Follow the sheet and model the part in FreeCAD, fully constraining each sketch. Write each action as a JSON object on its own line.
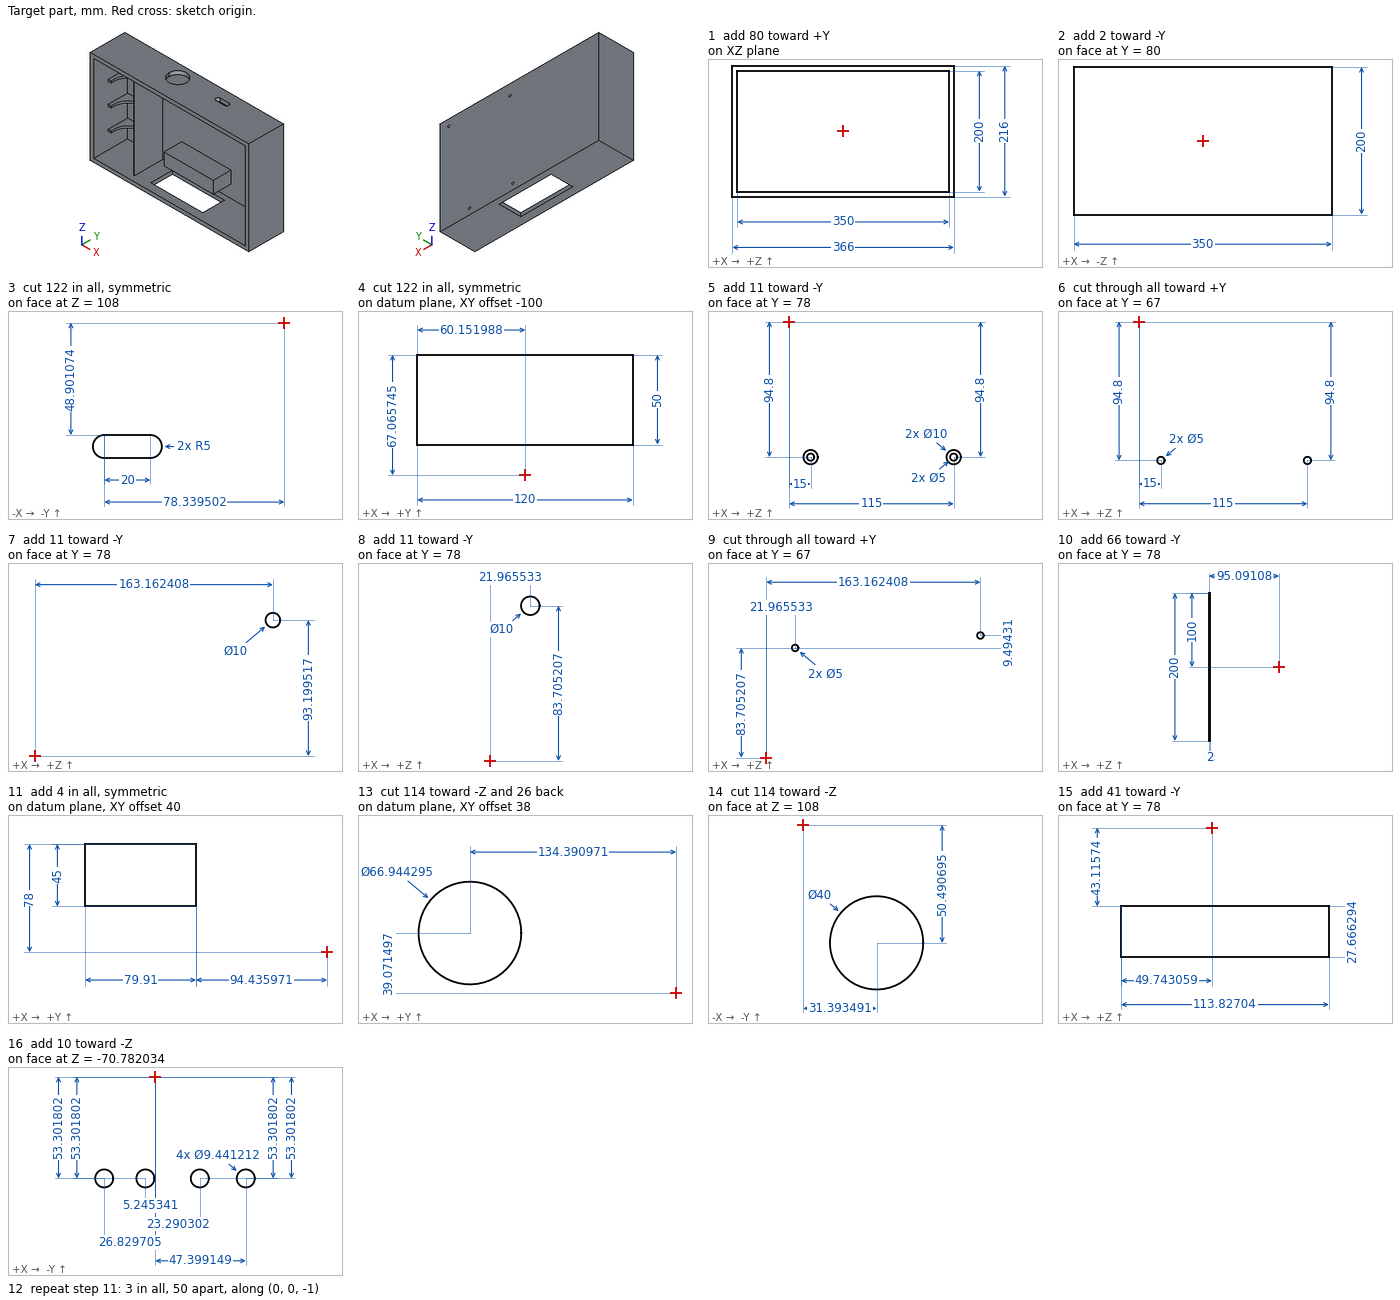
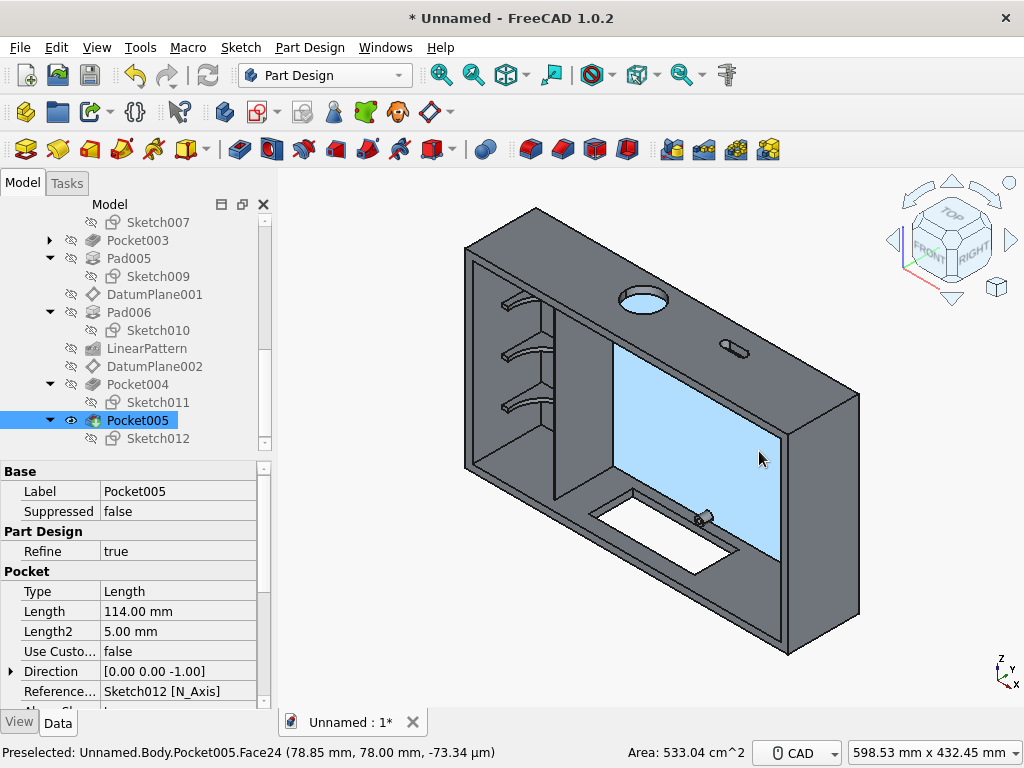
{"action": "left_click", "coordinate": [258, 112]}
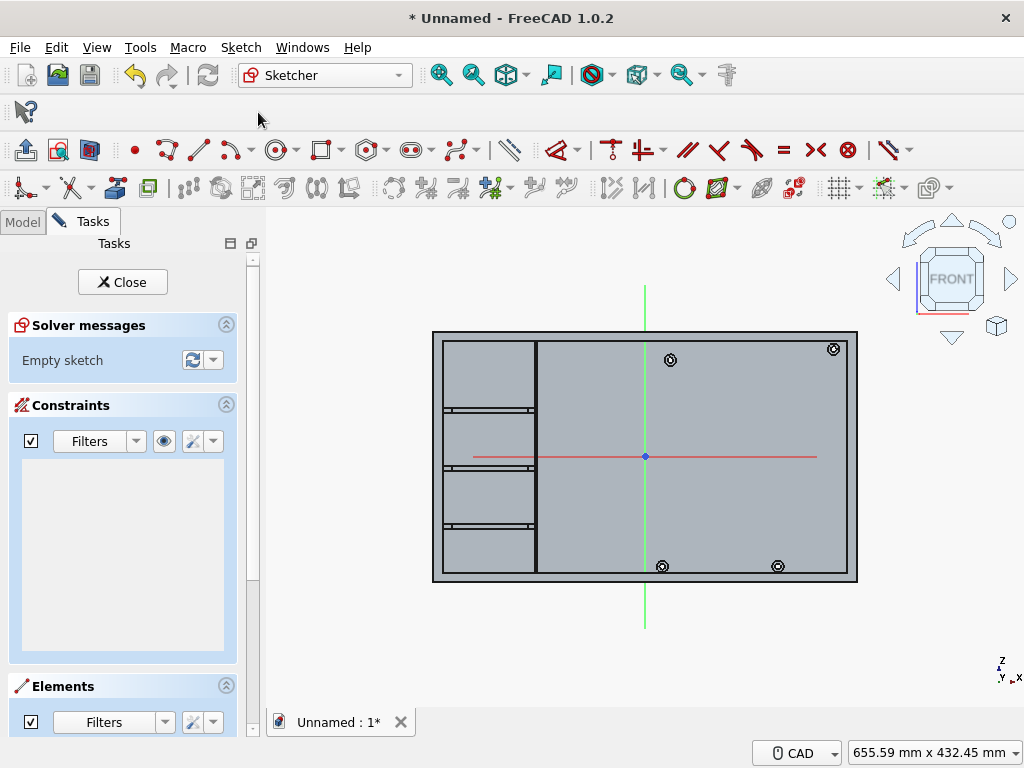
{"action": "key", "text": "q s"}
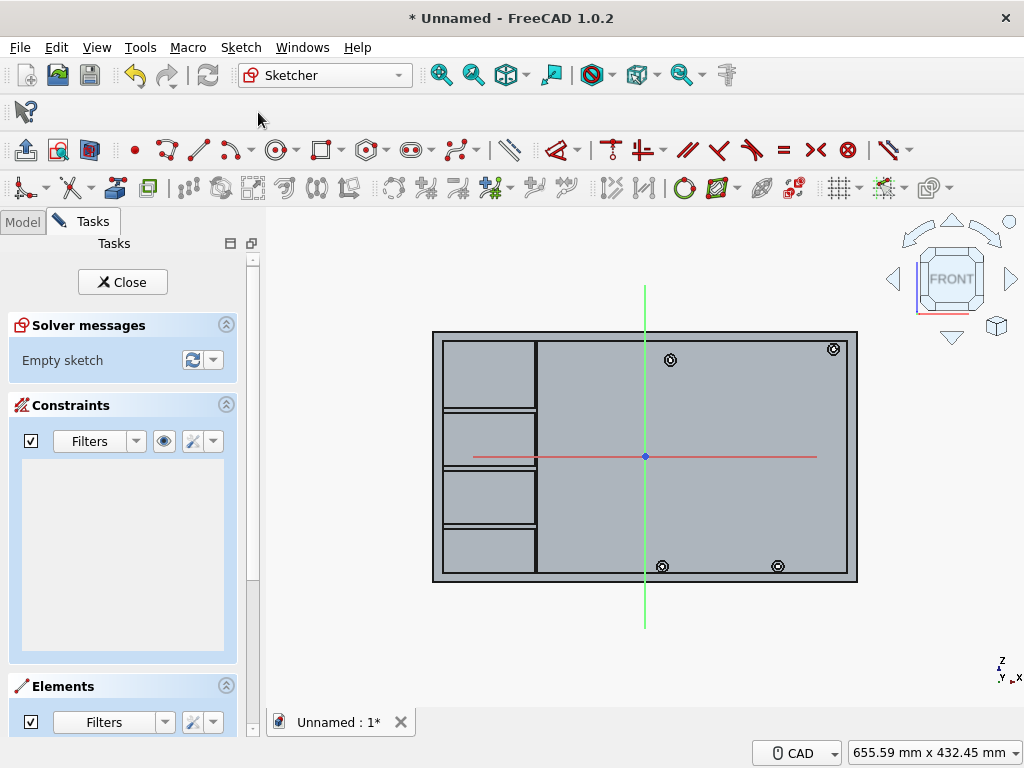
{"action": "scroll", "coordinate": [686, 516], "scroll_direction": "up", "scroll_amount": 6}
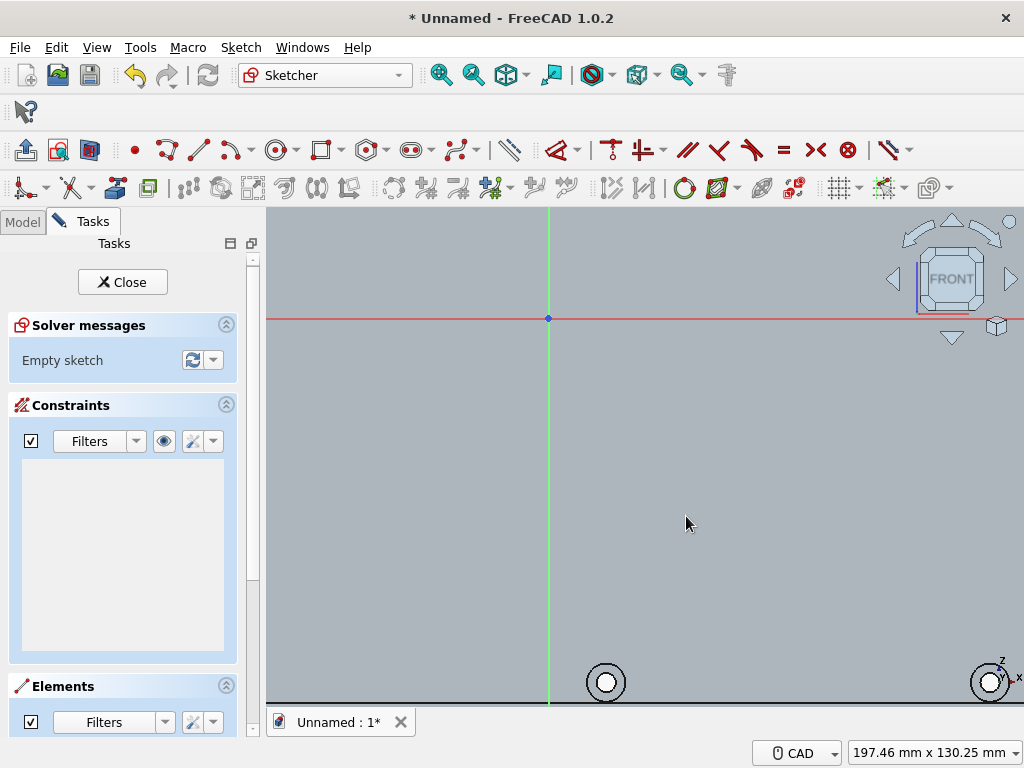
{"action": "key", "text": "g r"}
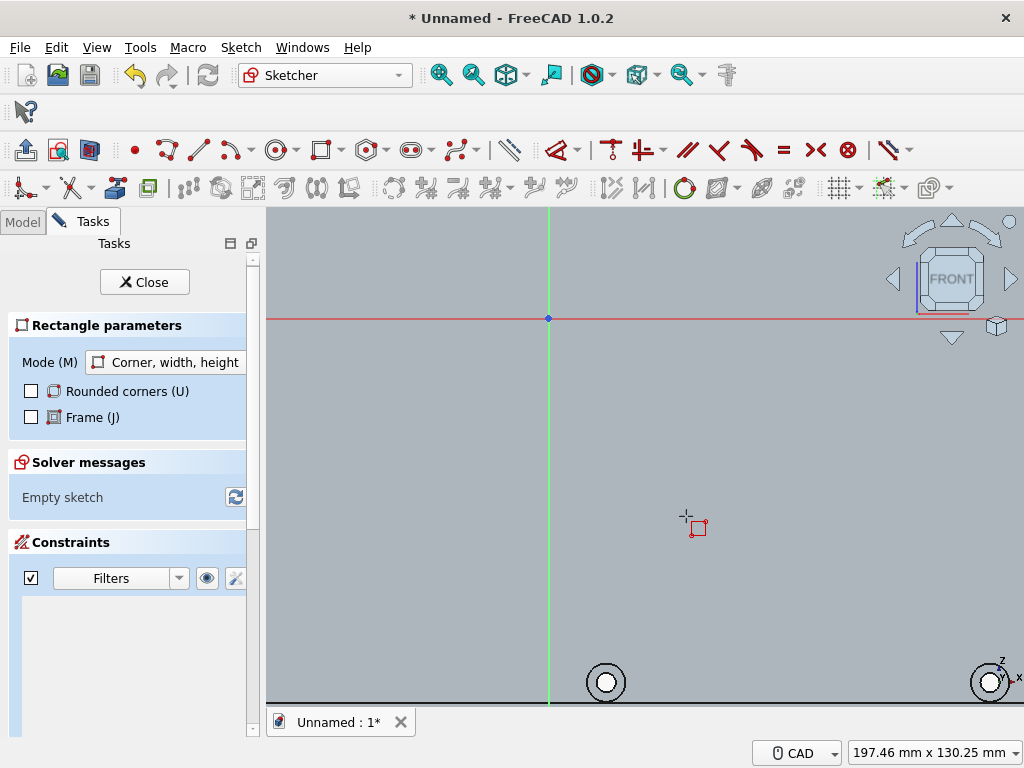
{"action": "left_click", "coordinate": [358, 484]}
{"action": "mouse_move", "coordinate": [795, 590]}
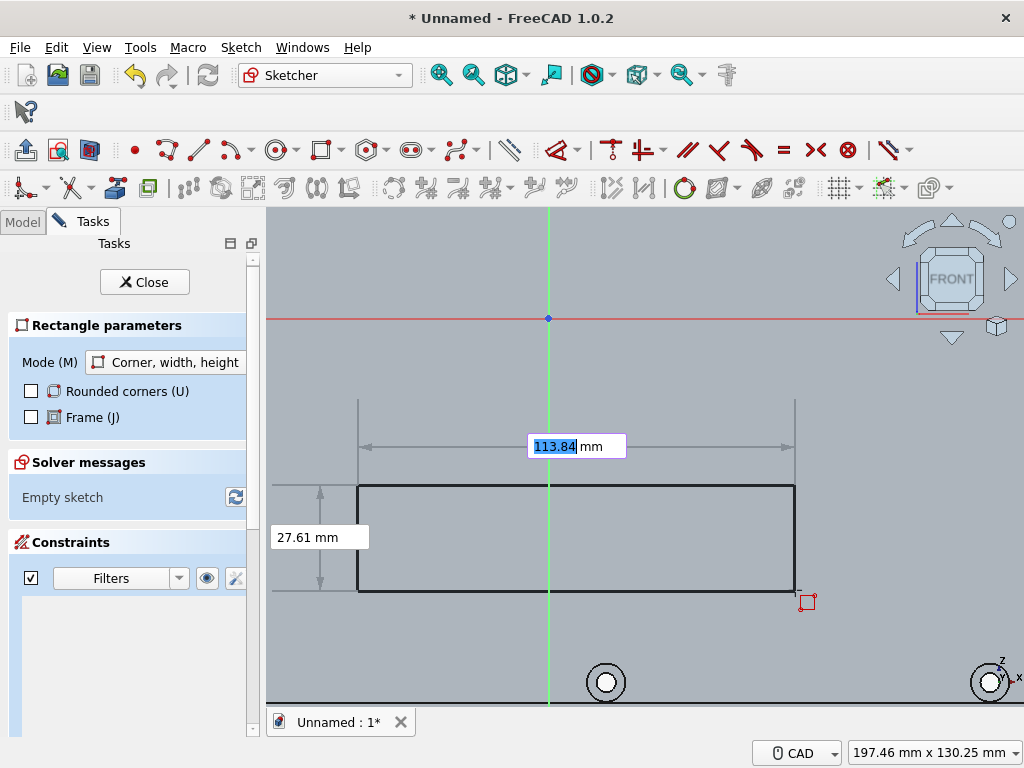
{"action": "type", "text": "113.82704"}
{"action": "key", "text": "Tab"}
{"action": "type", "text": "27.666294"}
{"action": "key", "text": "Return"}
{"action": "key", "text": "Escape"}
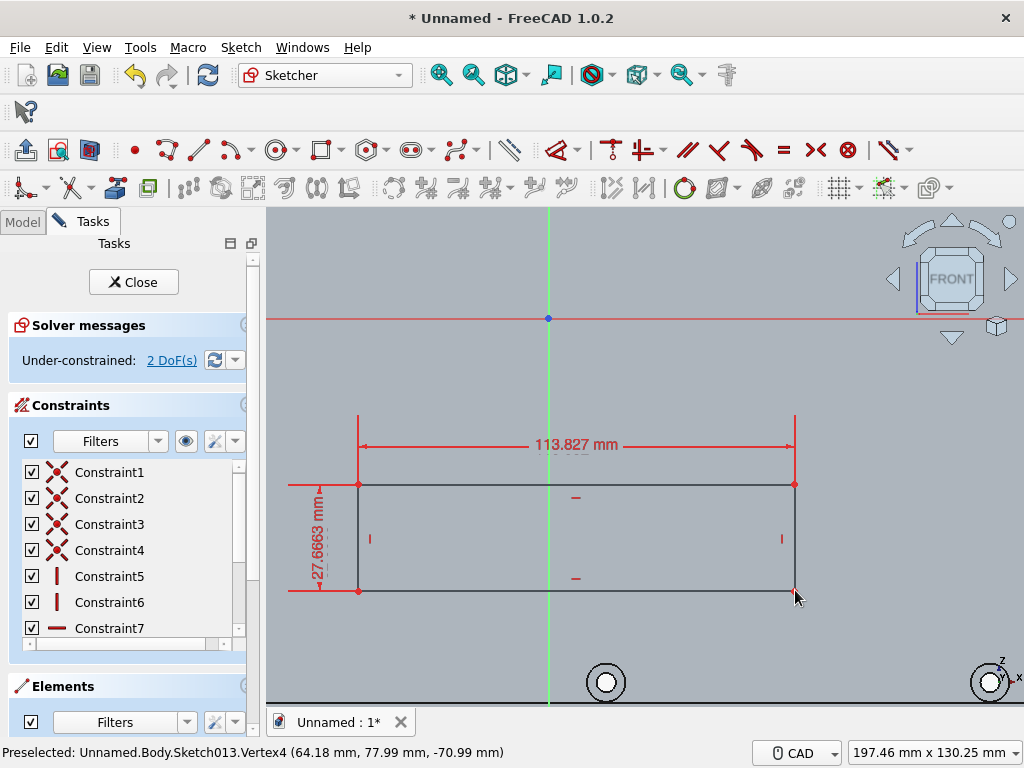
{"action": "key", "text": "d"}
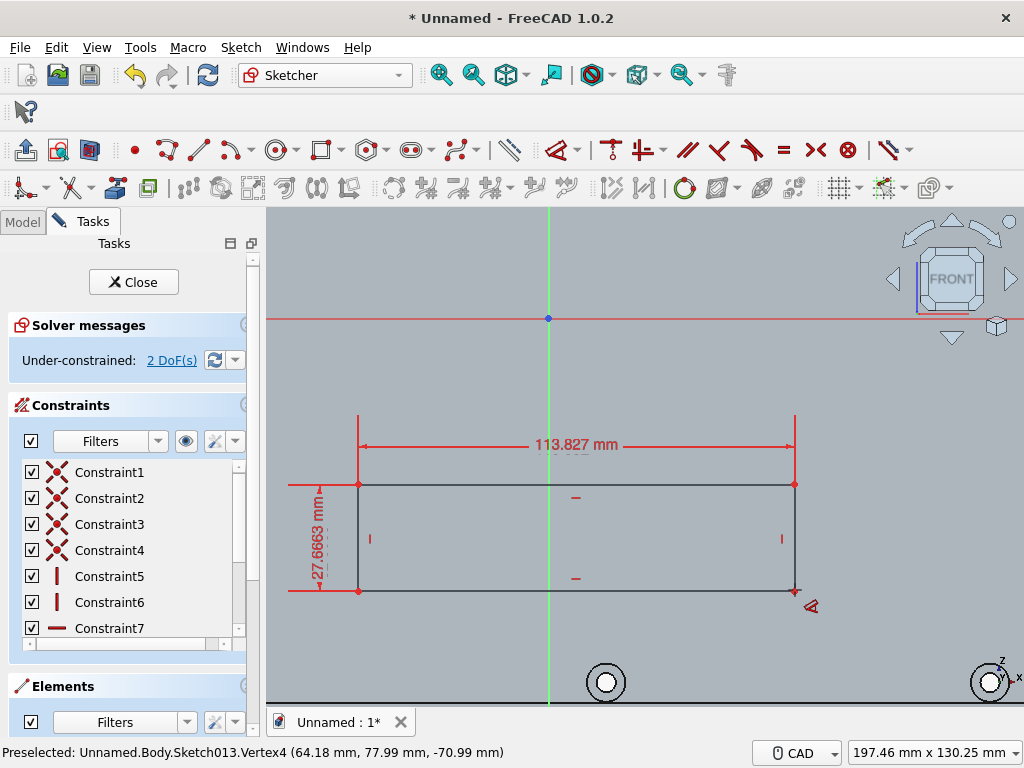
{"action": "left_click", "coordinate": [358, 485]}
{"action": "left_click", "coordinate": [324, 402]}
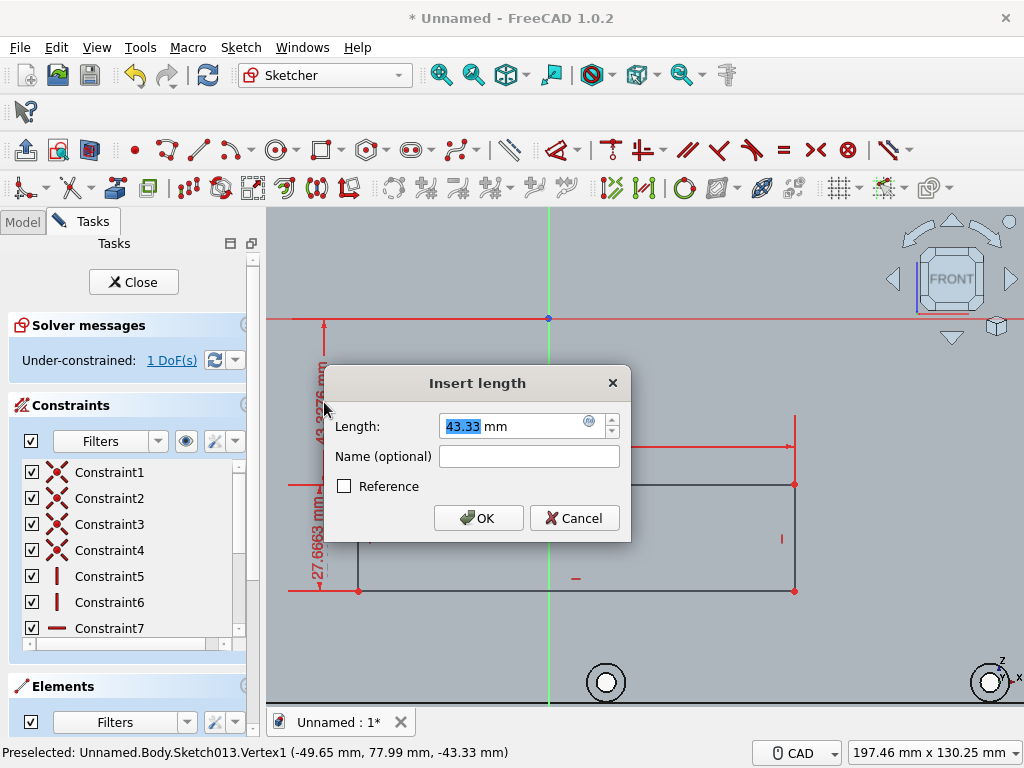
{"action": "type", "text": "43.11574"}
{"action": "key", "text": "Return"}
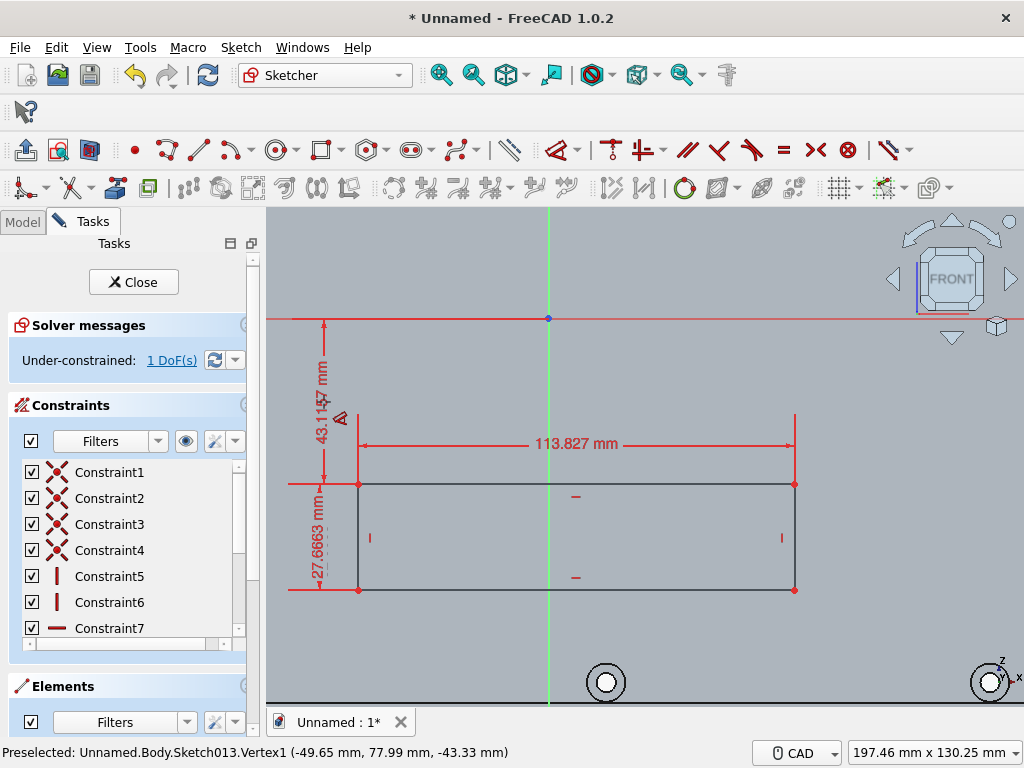
{"action": "left_click", "coordinate": [358, 484]}
{"action": "left_click", "coordinate": [453, 285]}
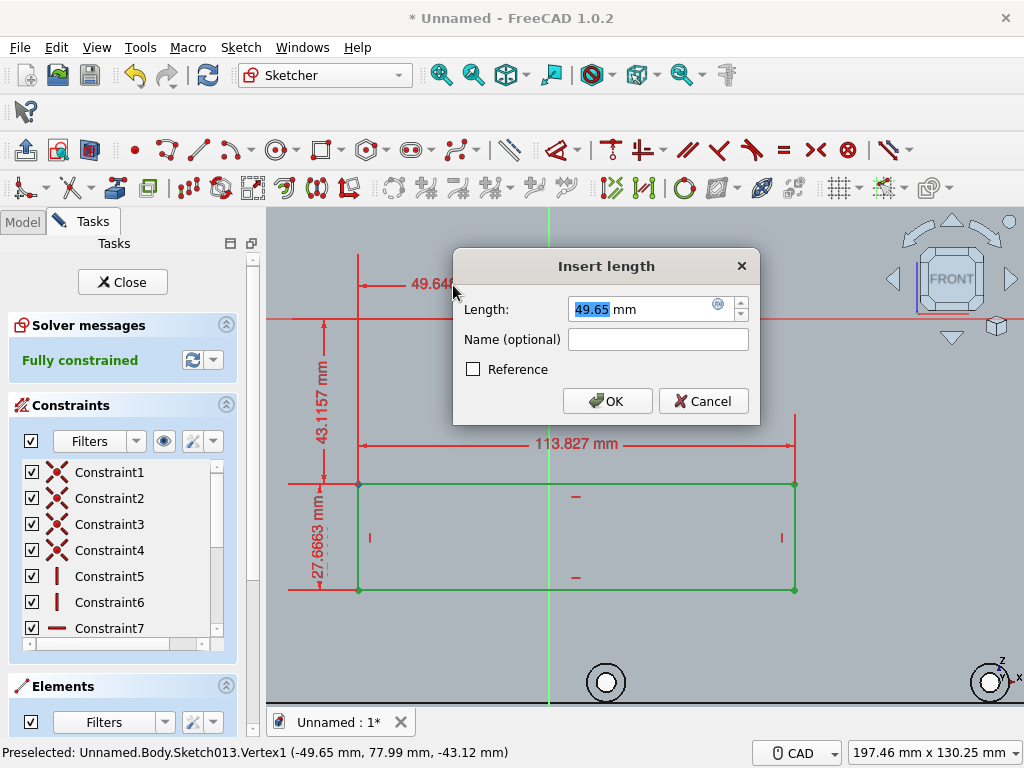
{"action": "type", "text": "49.743059"}
{"action": "key", "text": "Return"}
{"action": "key", "text": "Escape"}